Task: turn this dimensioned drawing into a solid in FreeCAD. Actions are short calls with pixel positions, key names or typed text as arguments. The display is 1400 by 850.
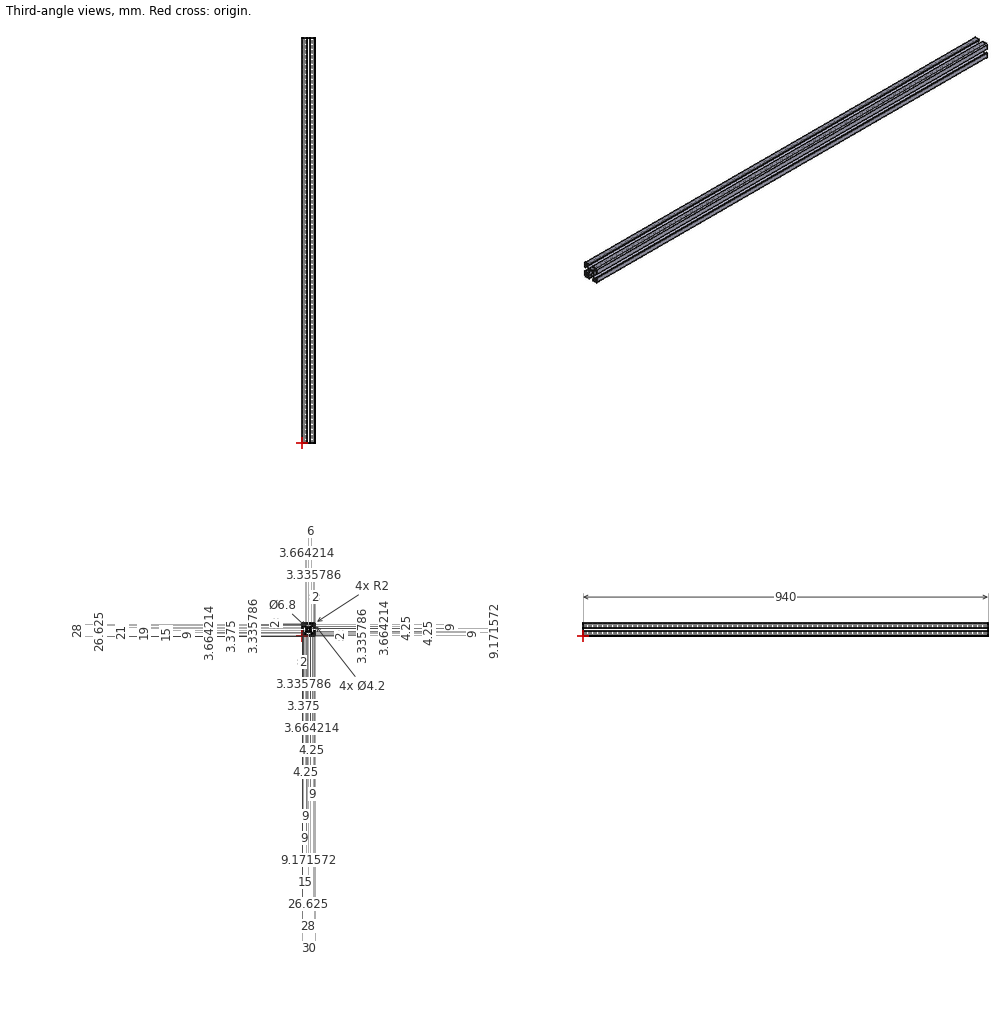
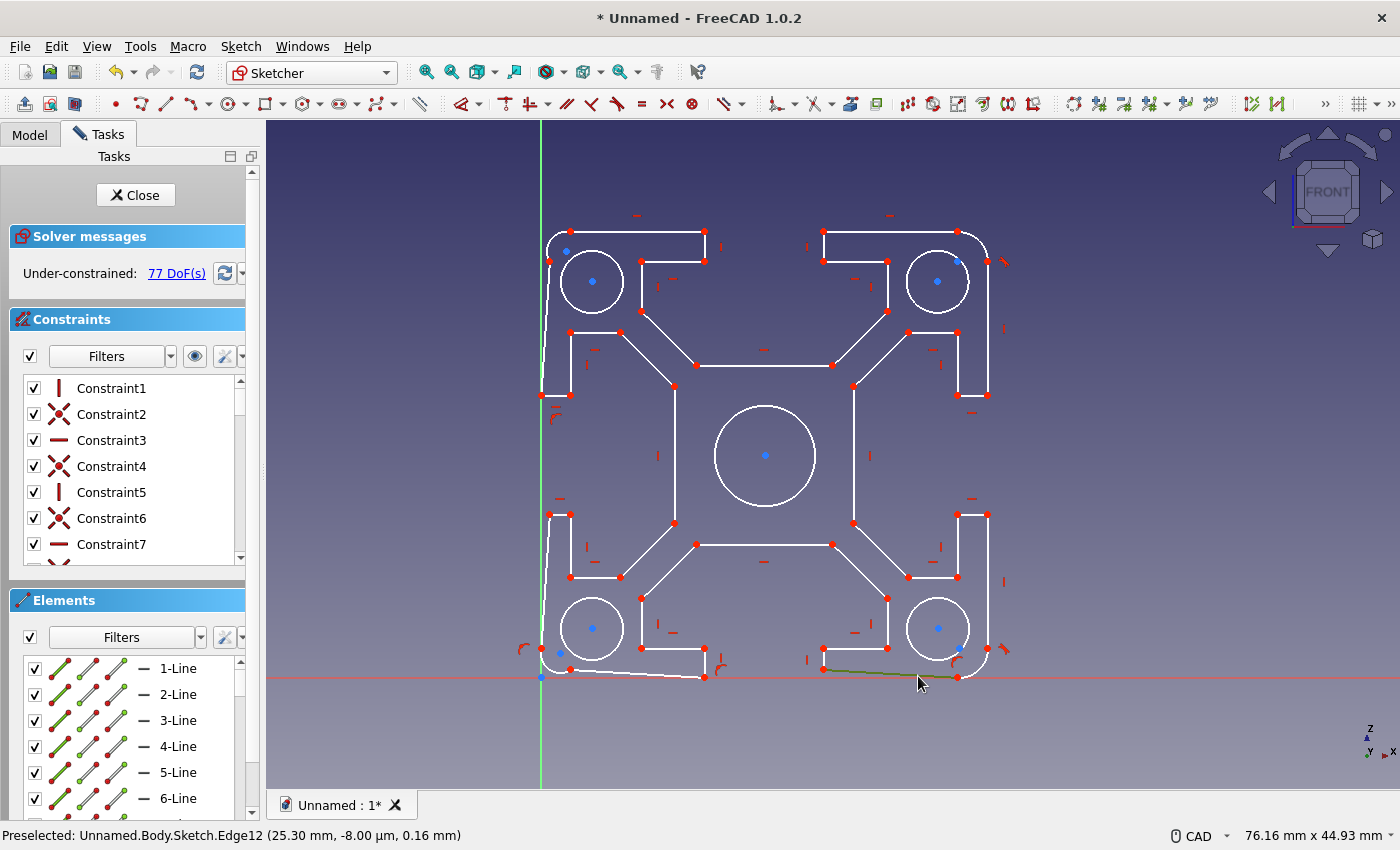
click(971, 675)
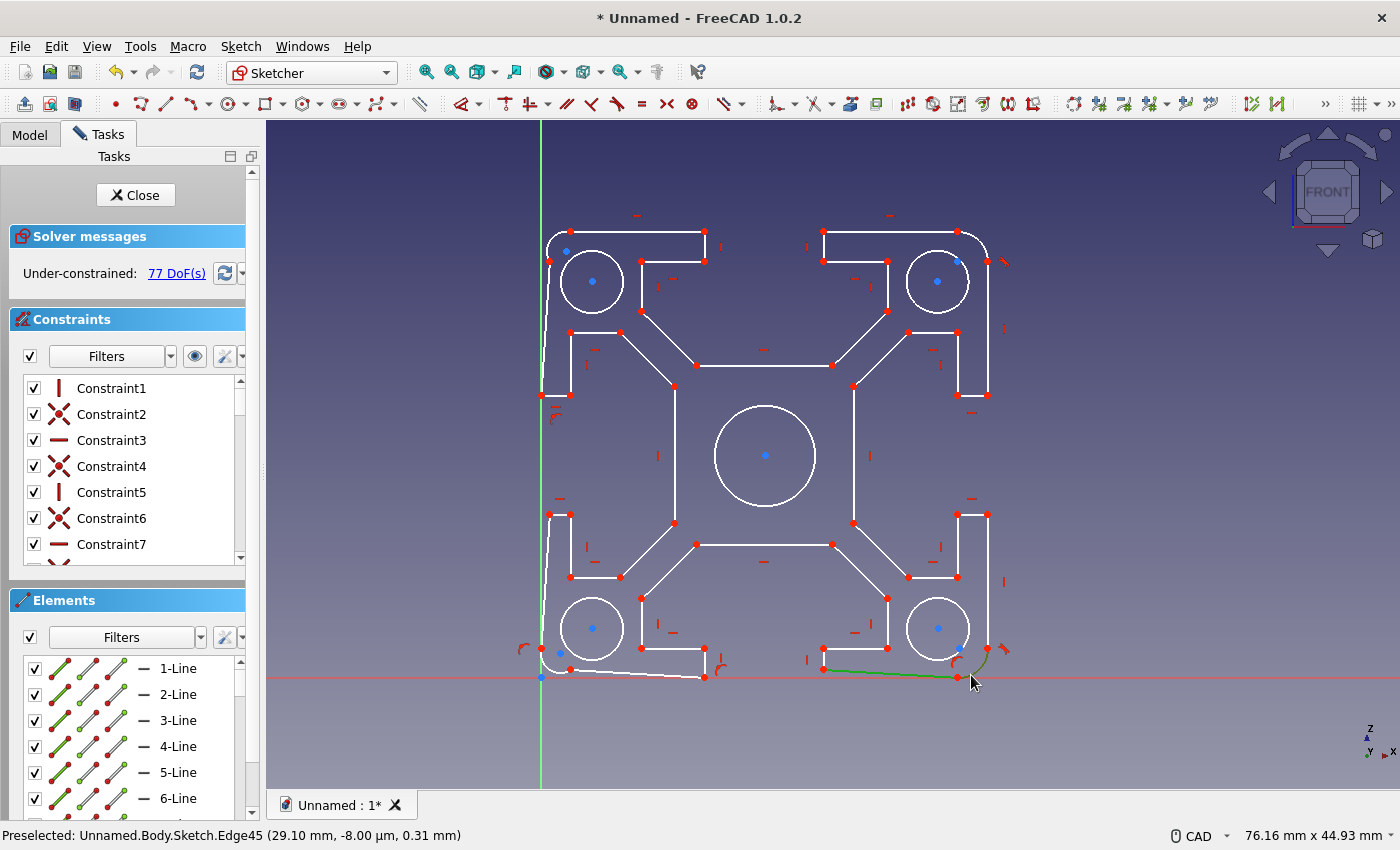
key(t)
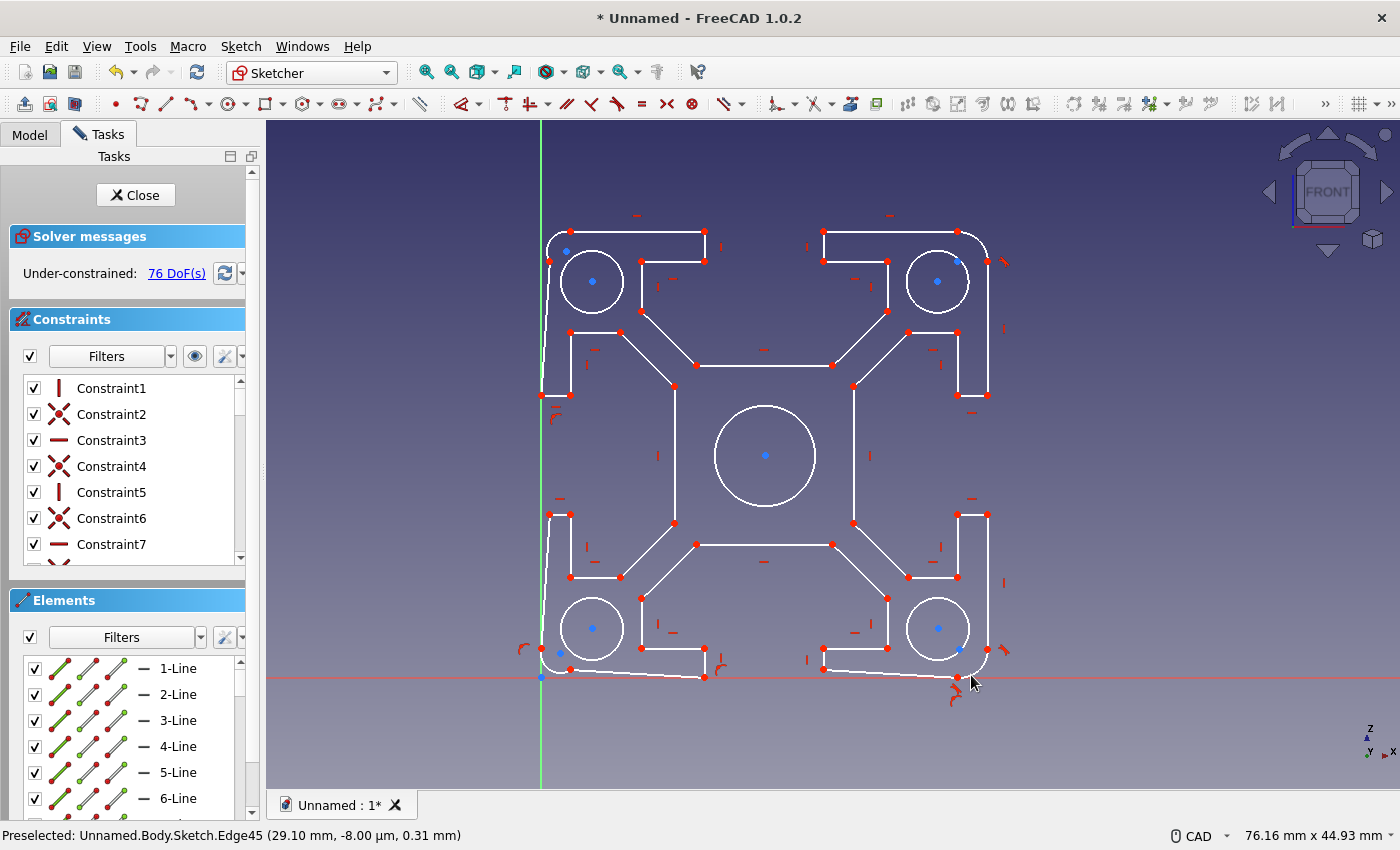
click(665, 676)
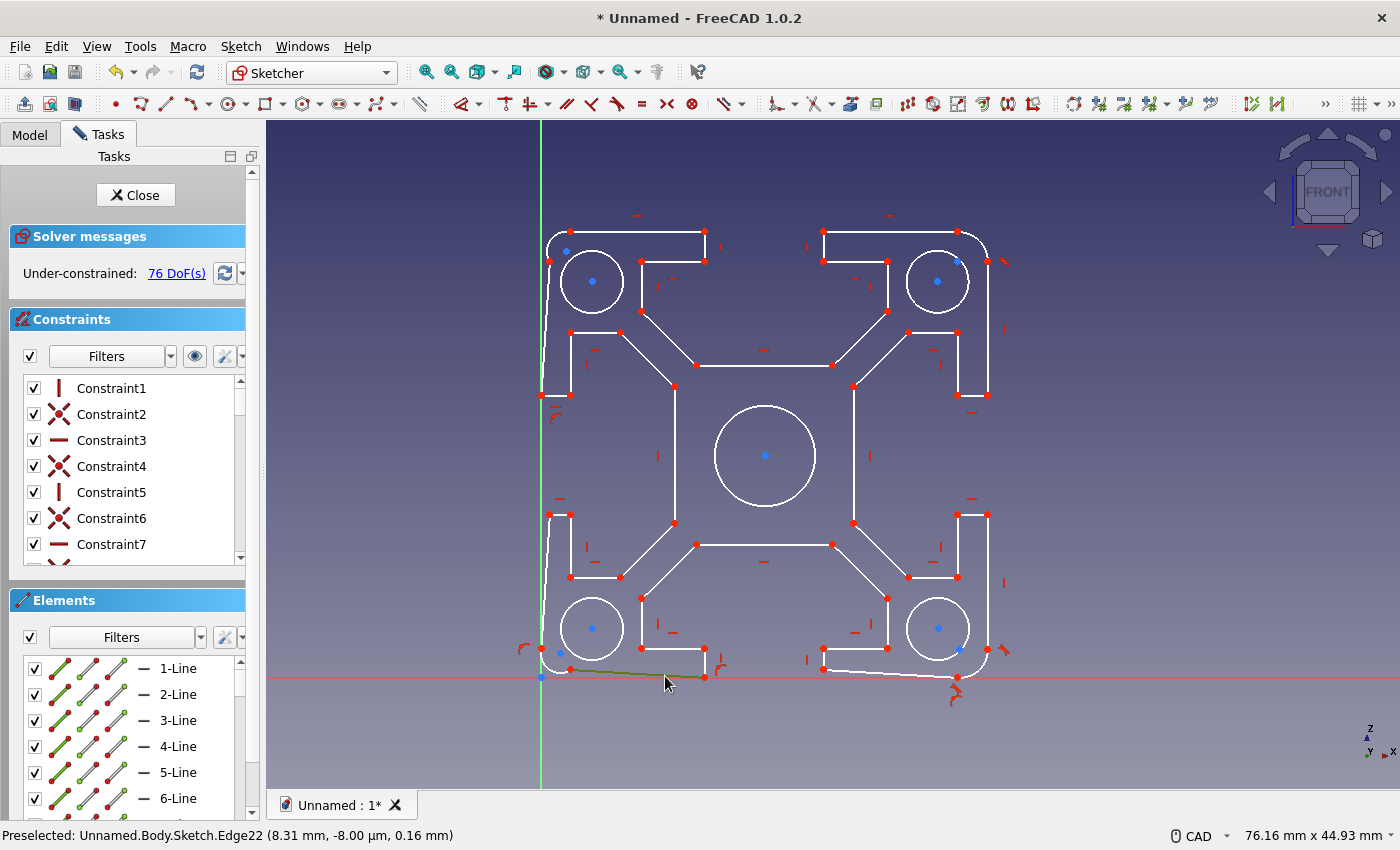
click(543, 662)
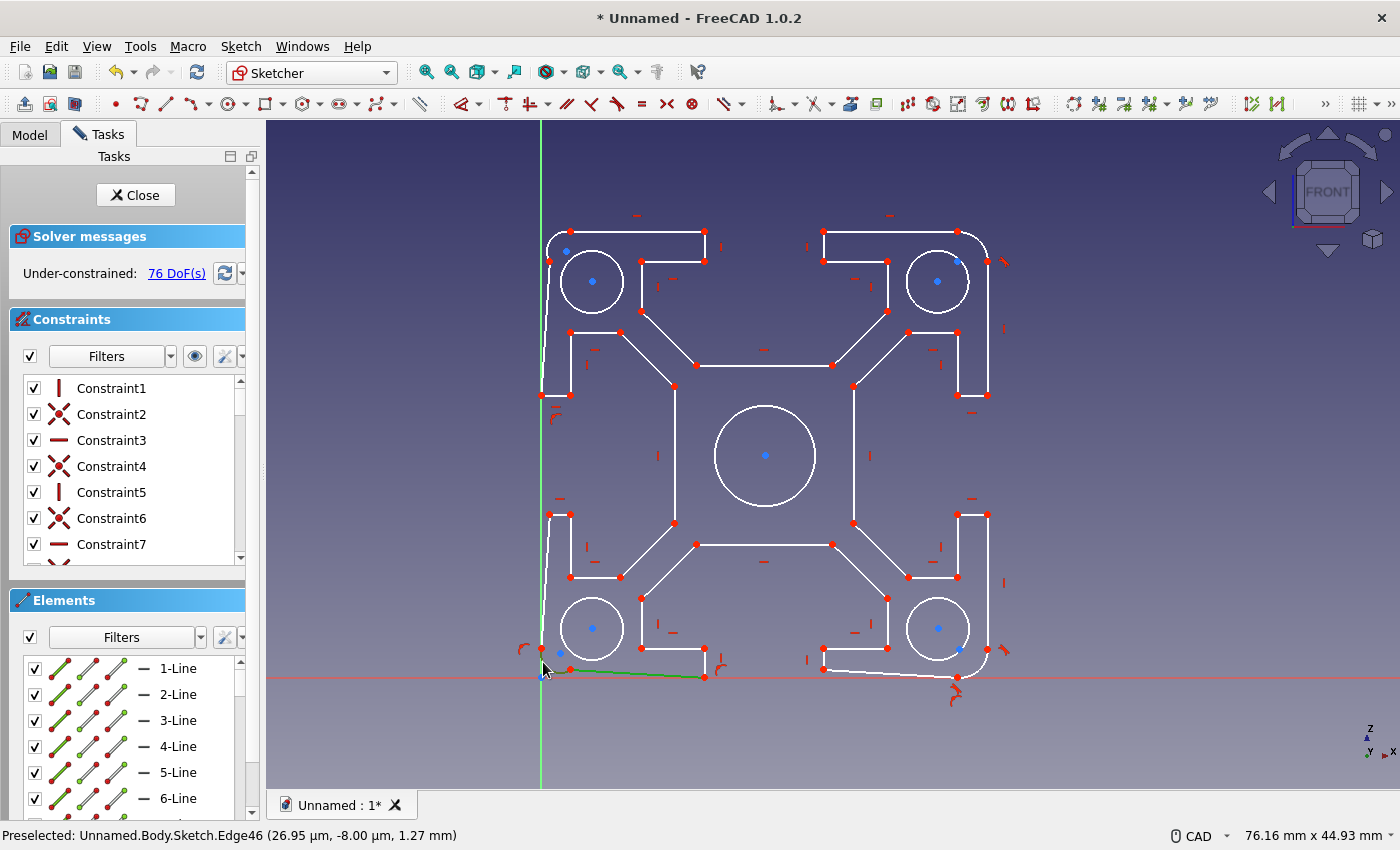
key(t)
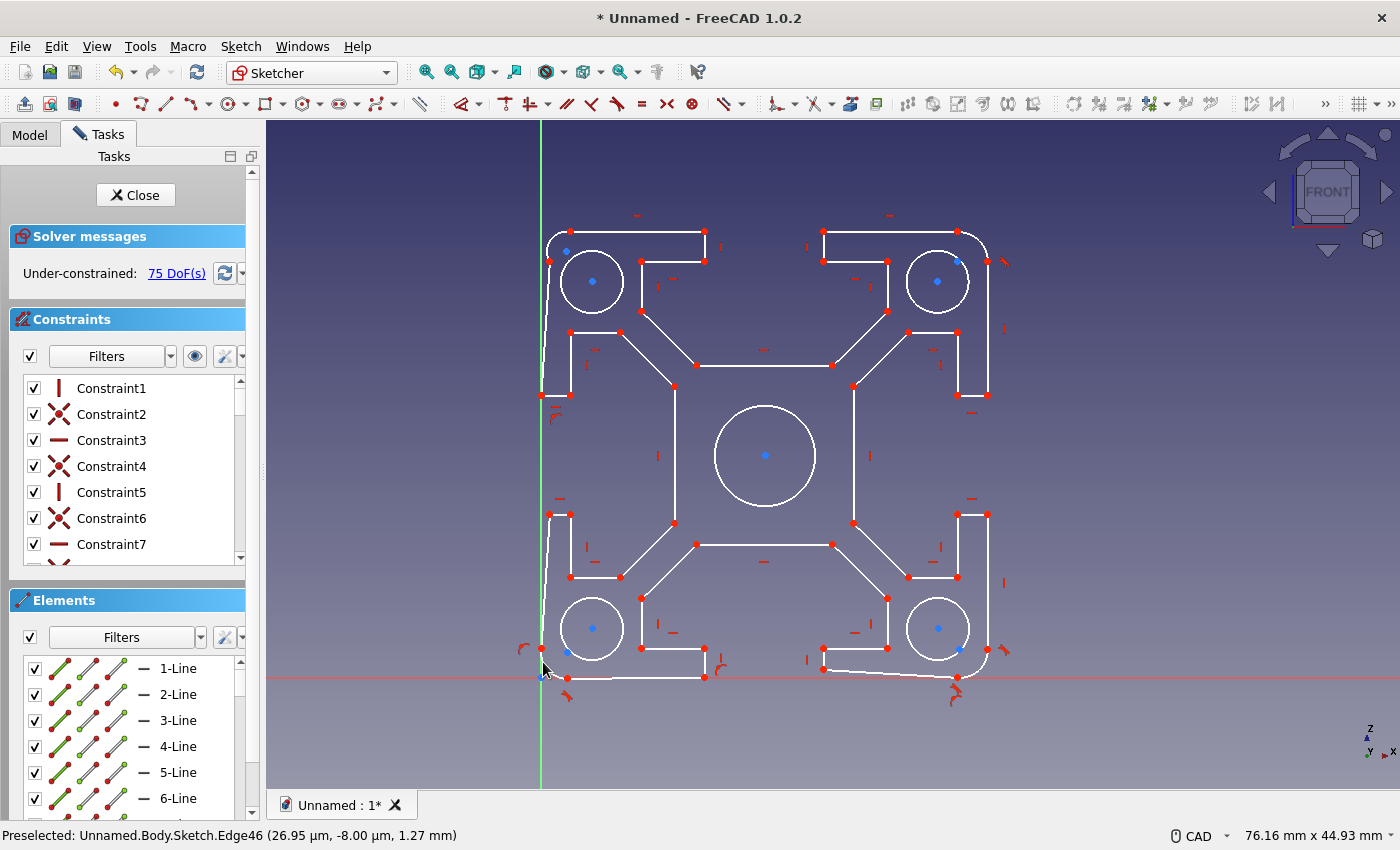
click(544, 609)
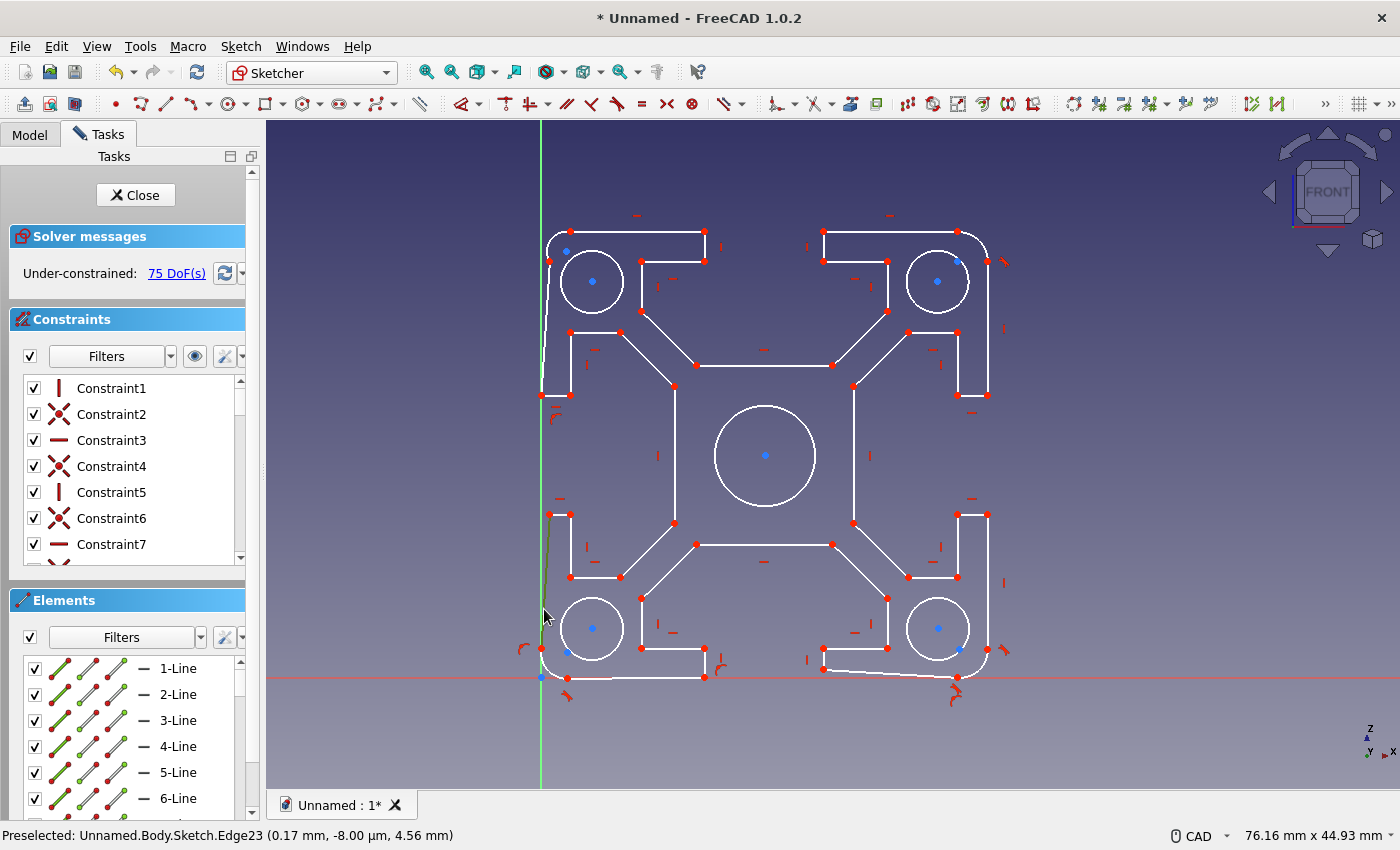
click(543, 662)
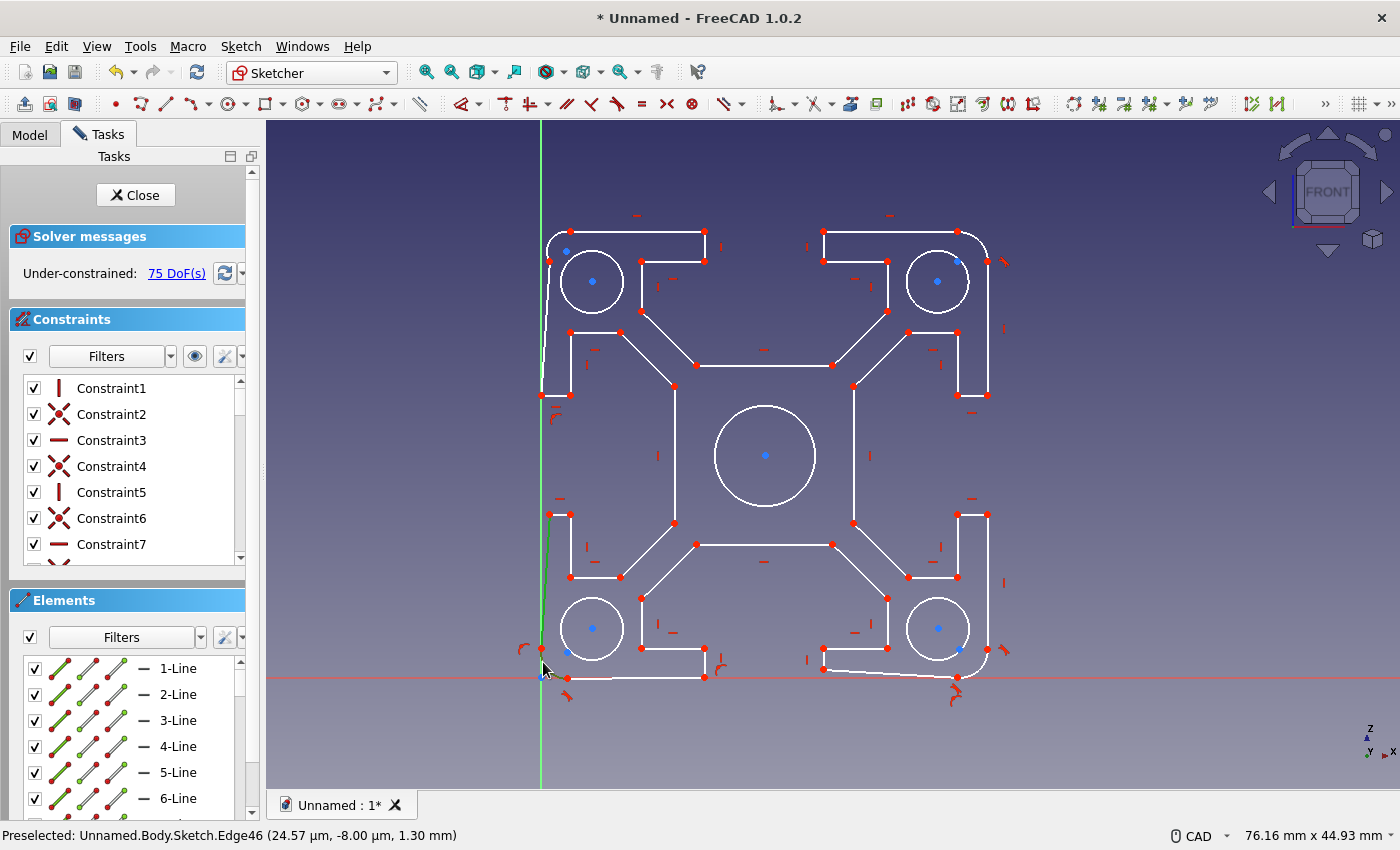
key(t)